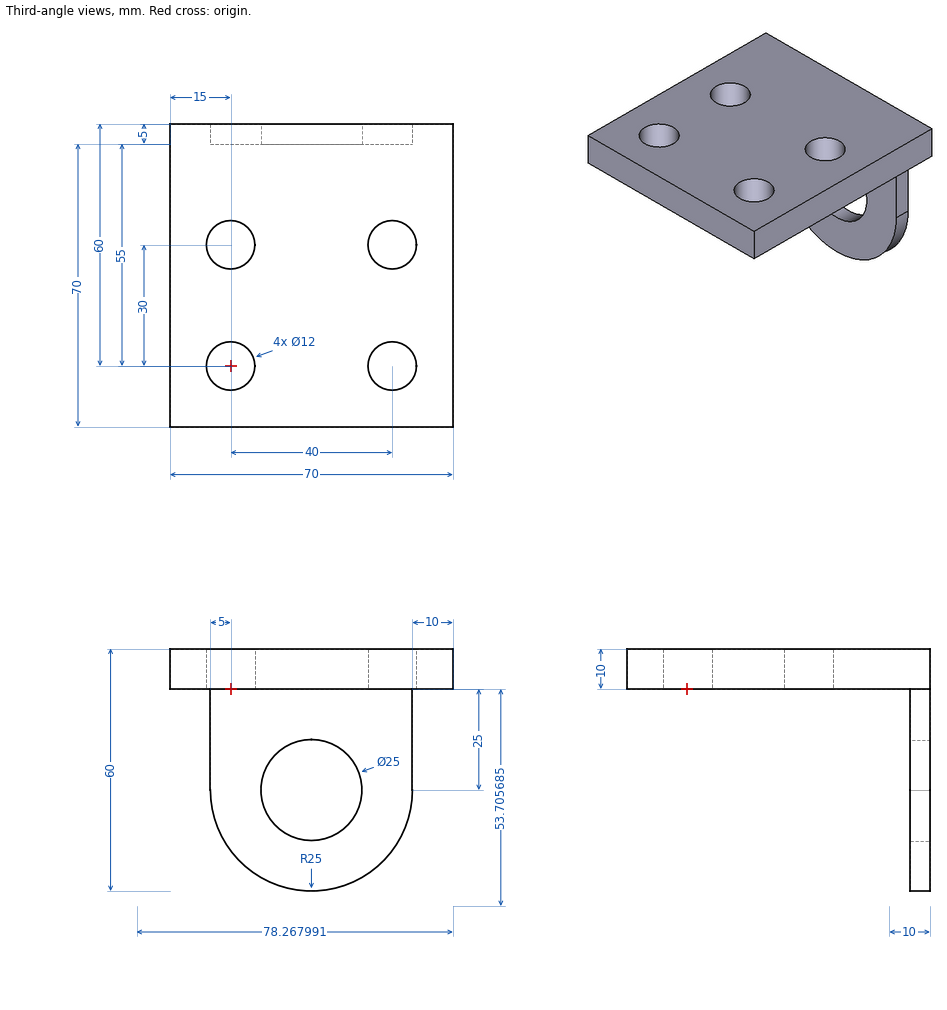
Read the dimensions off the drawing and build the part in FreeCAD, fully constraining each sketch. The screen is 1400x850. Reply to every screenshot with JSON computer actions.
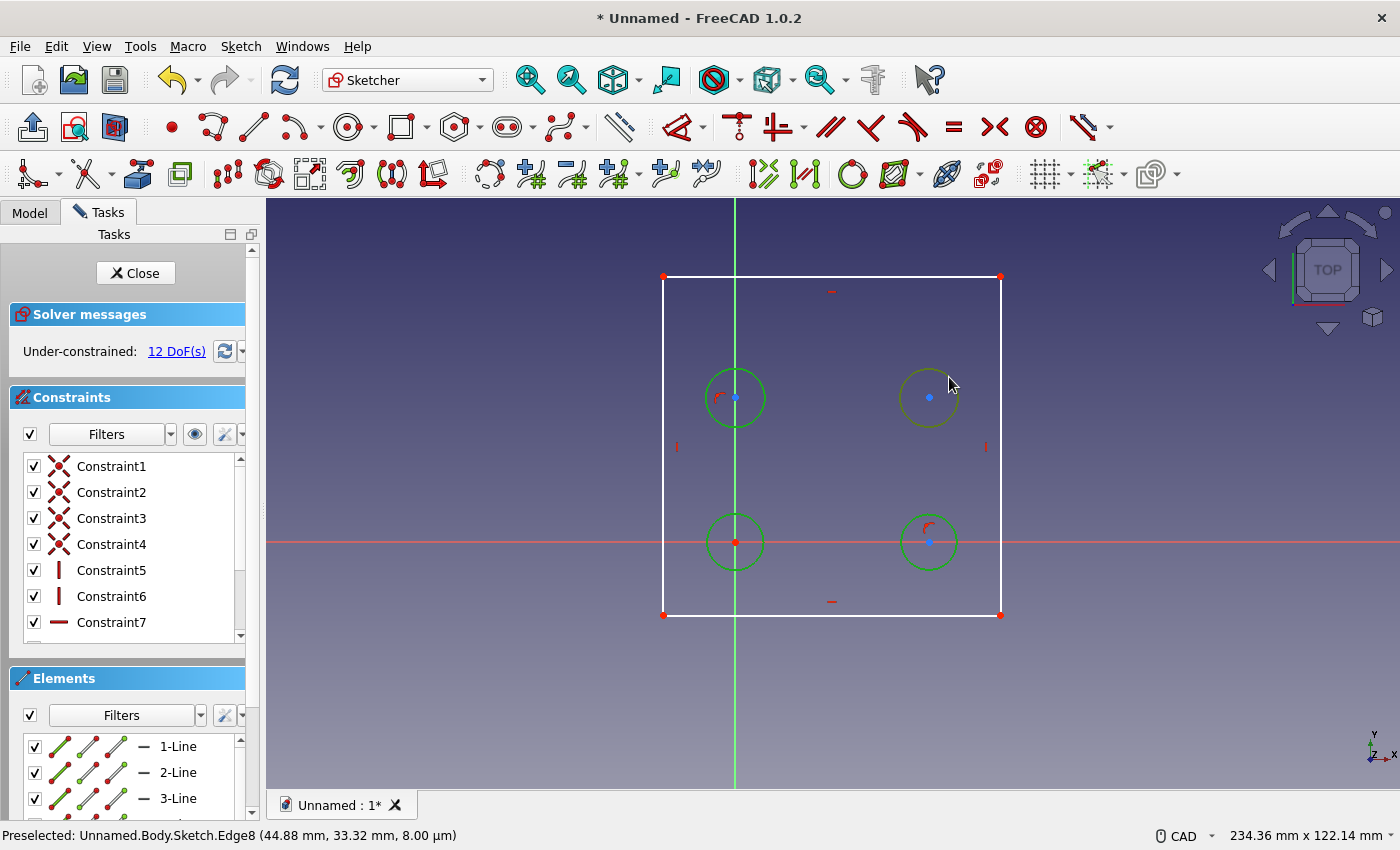
{"action": "left_click", "coordinate": [954, 128]}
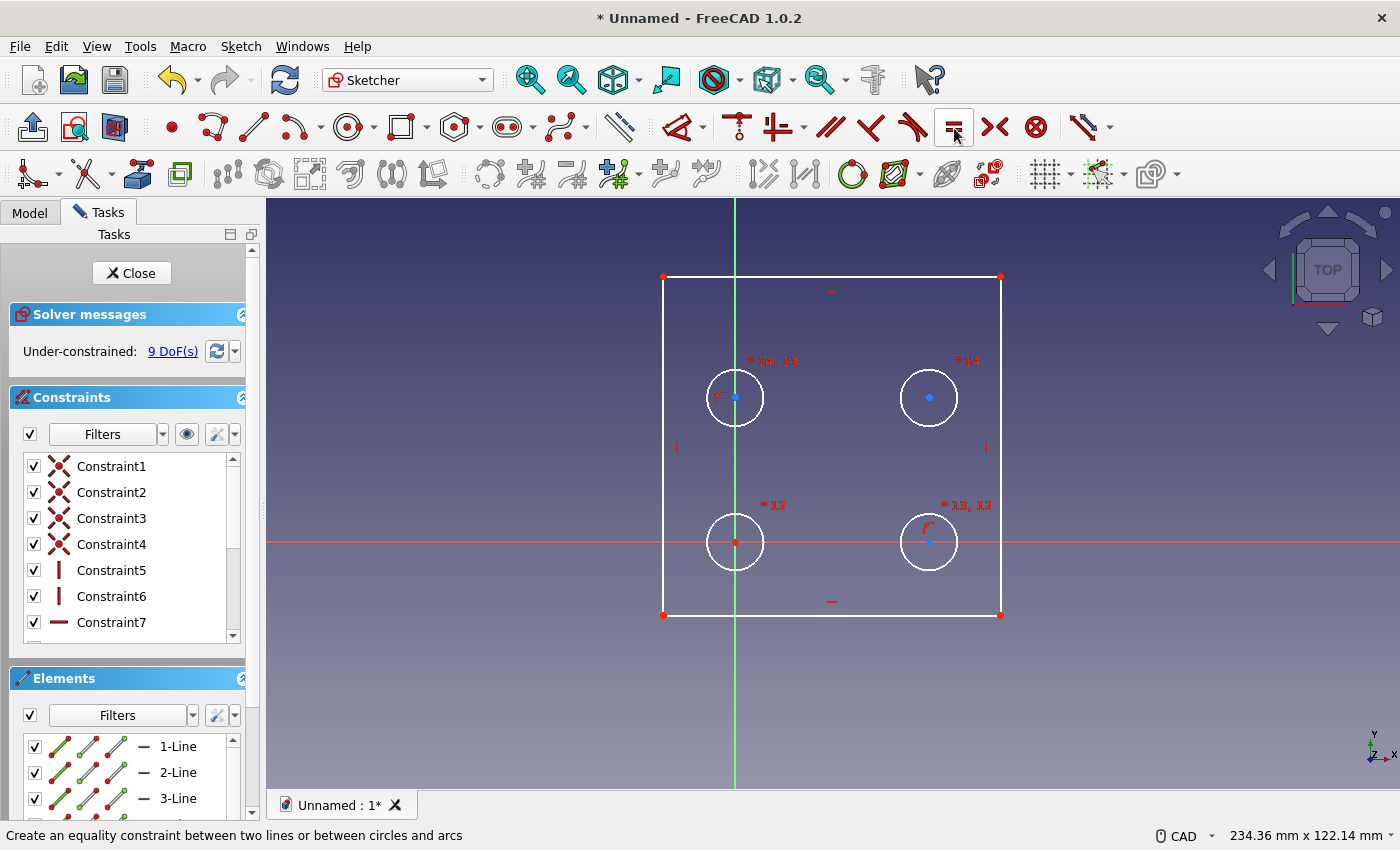
{"action": "left_click", "coordinate": [676, 128]}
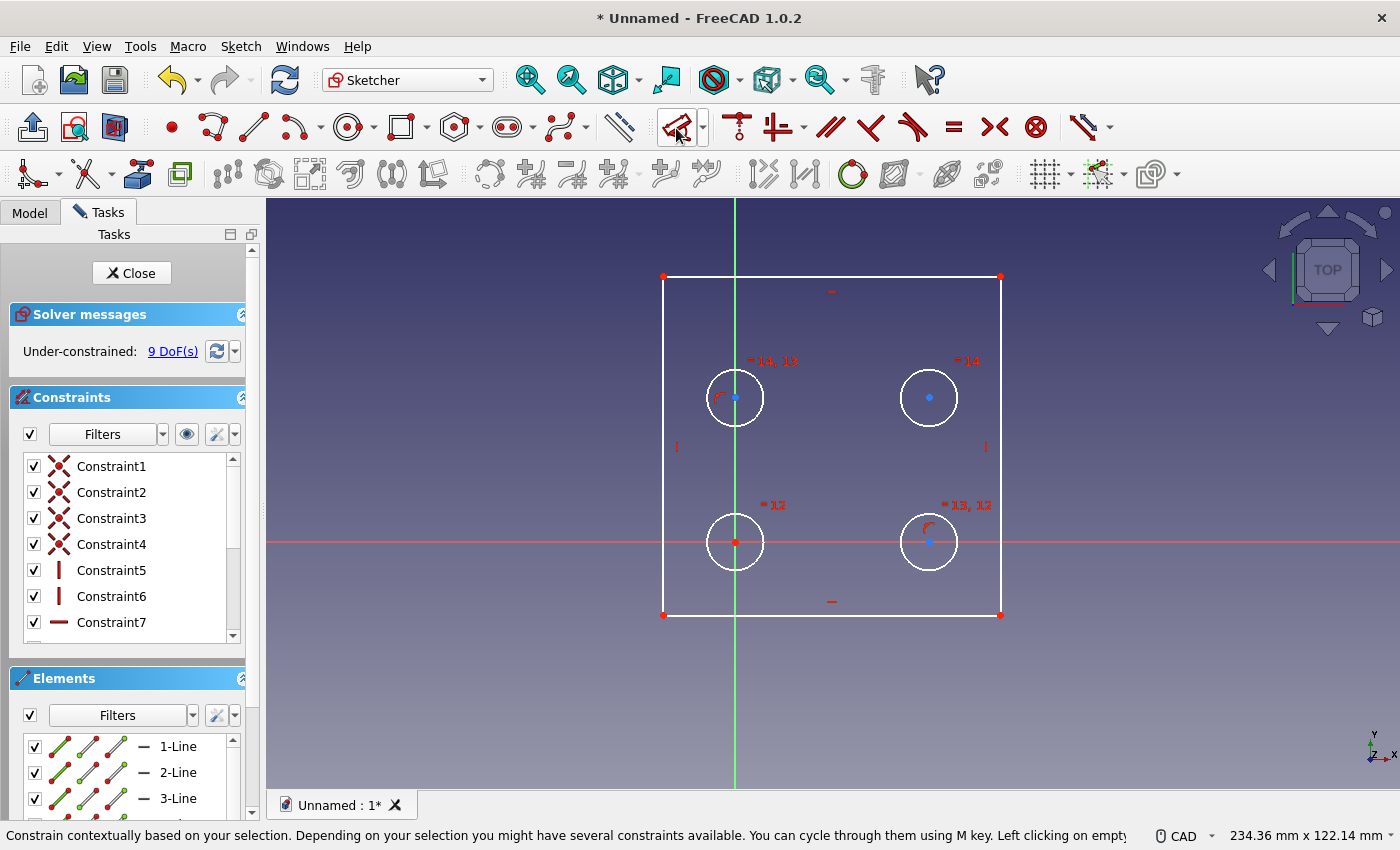
{"action": "left_click", "coordinate": [755, 522]}
{"action": "left_click", "coordinate": [777, 499]}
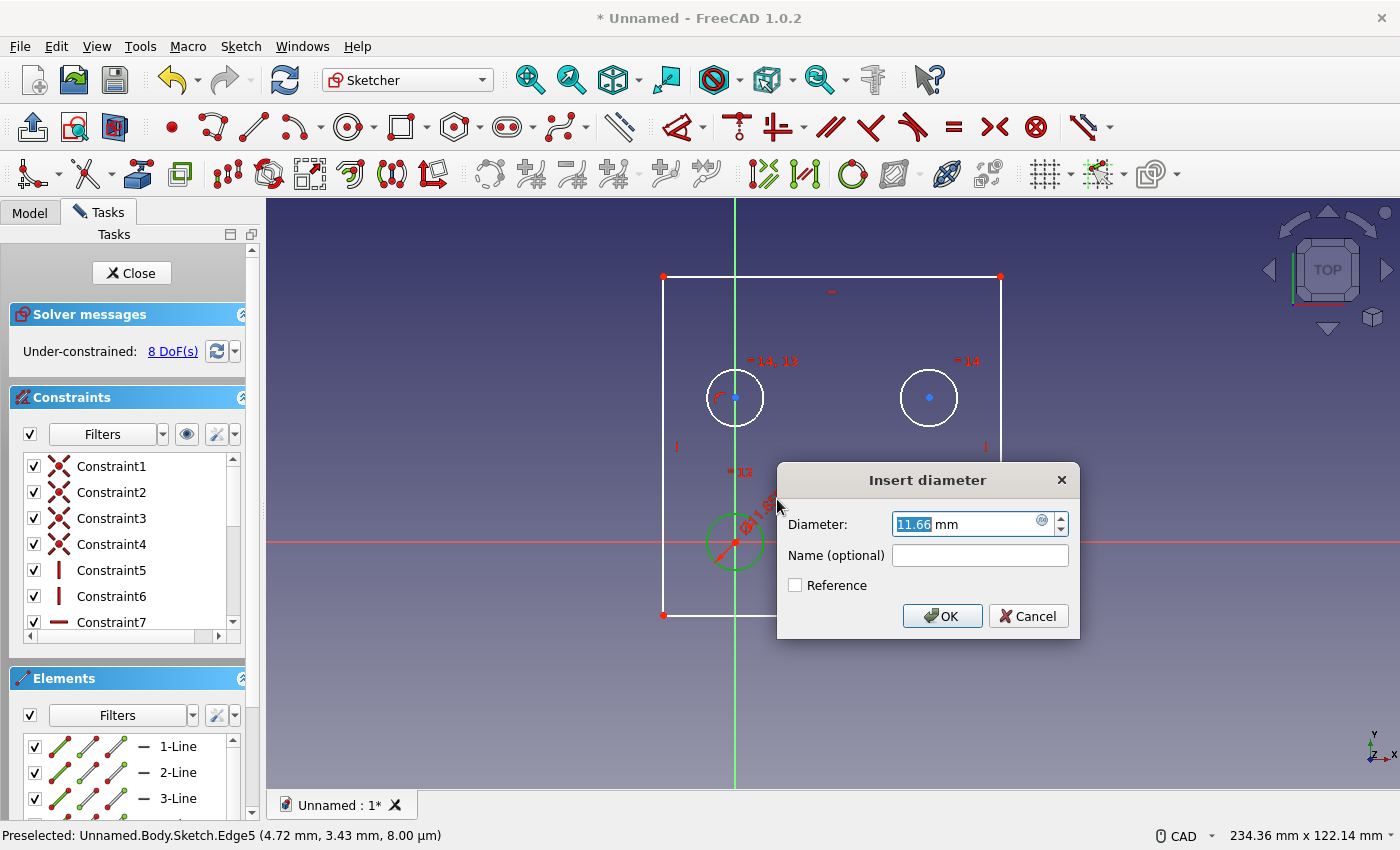
{"action": "type", "text": "12"}
{"action": "key", "text": "Return"}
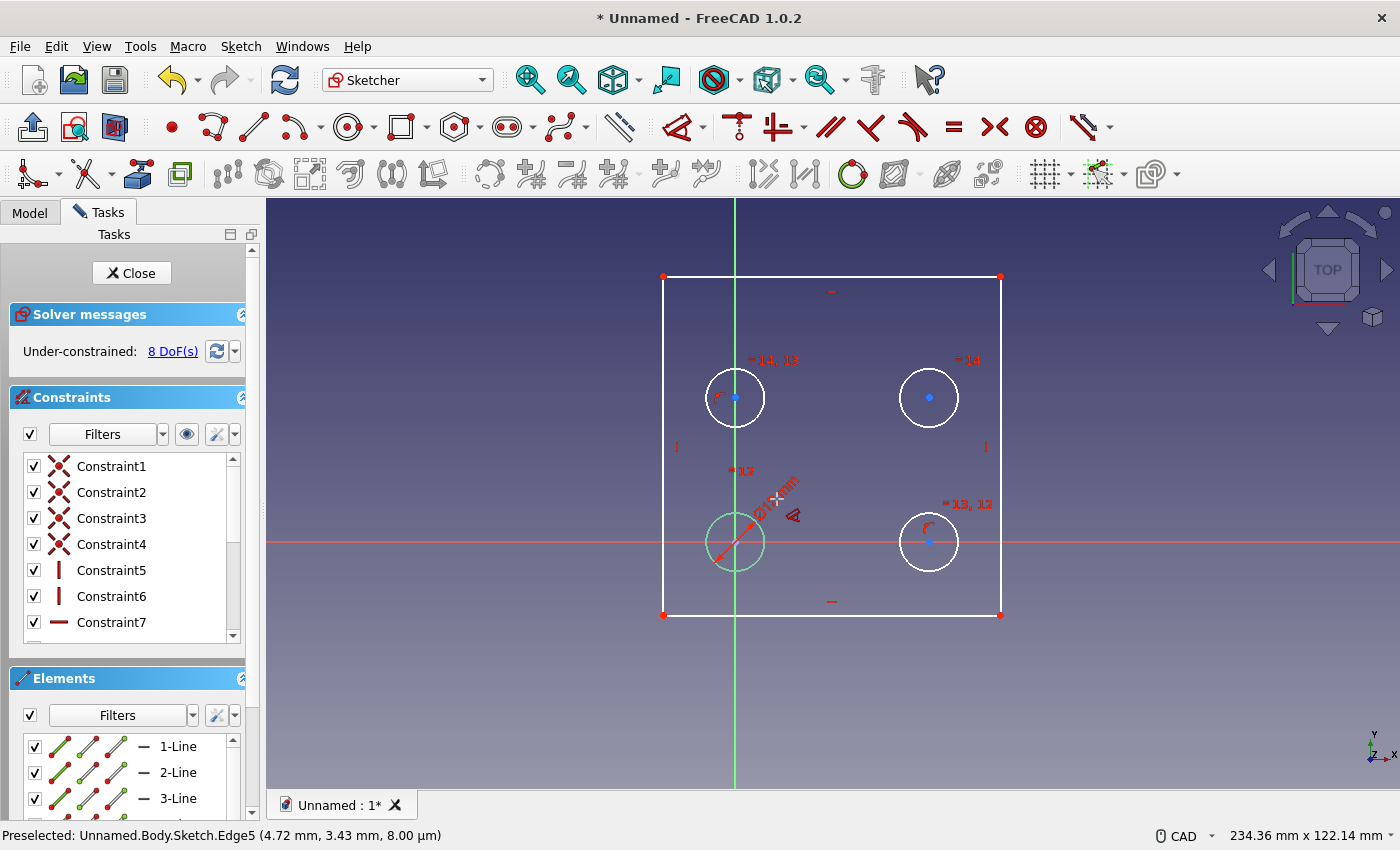
{"action": "left_click", "coordinate": [663, 379]}
{"action": "left_click", "coordinate": [629, 447]}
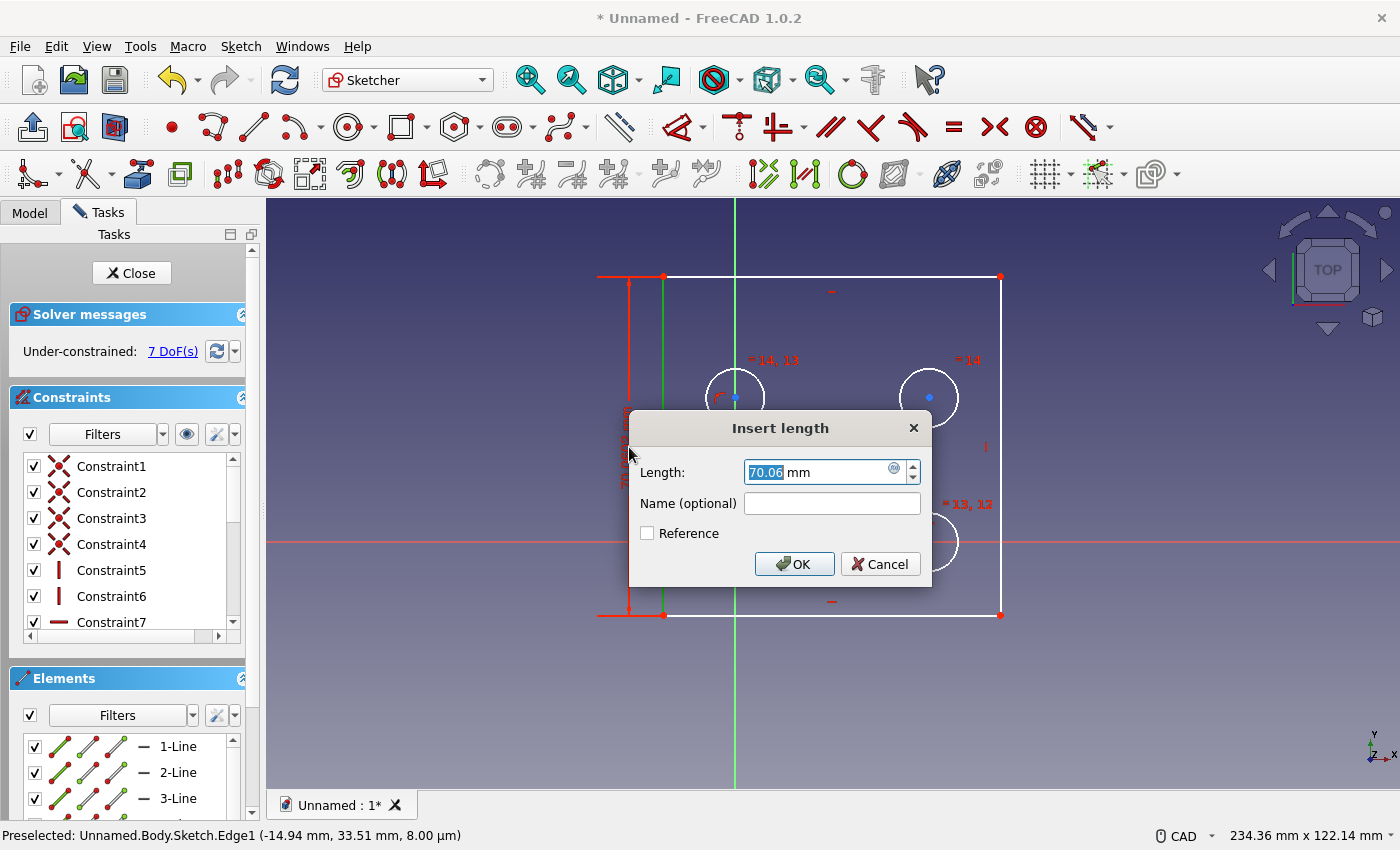
{"action": "type", "text": "70"}
{"action": "key", "text": "Return"}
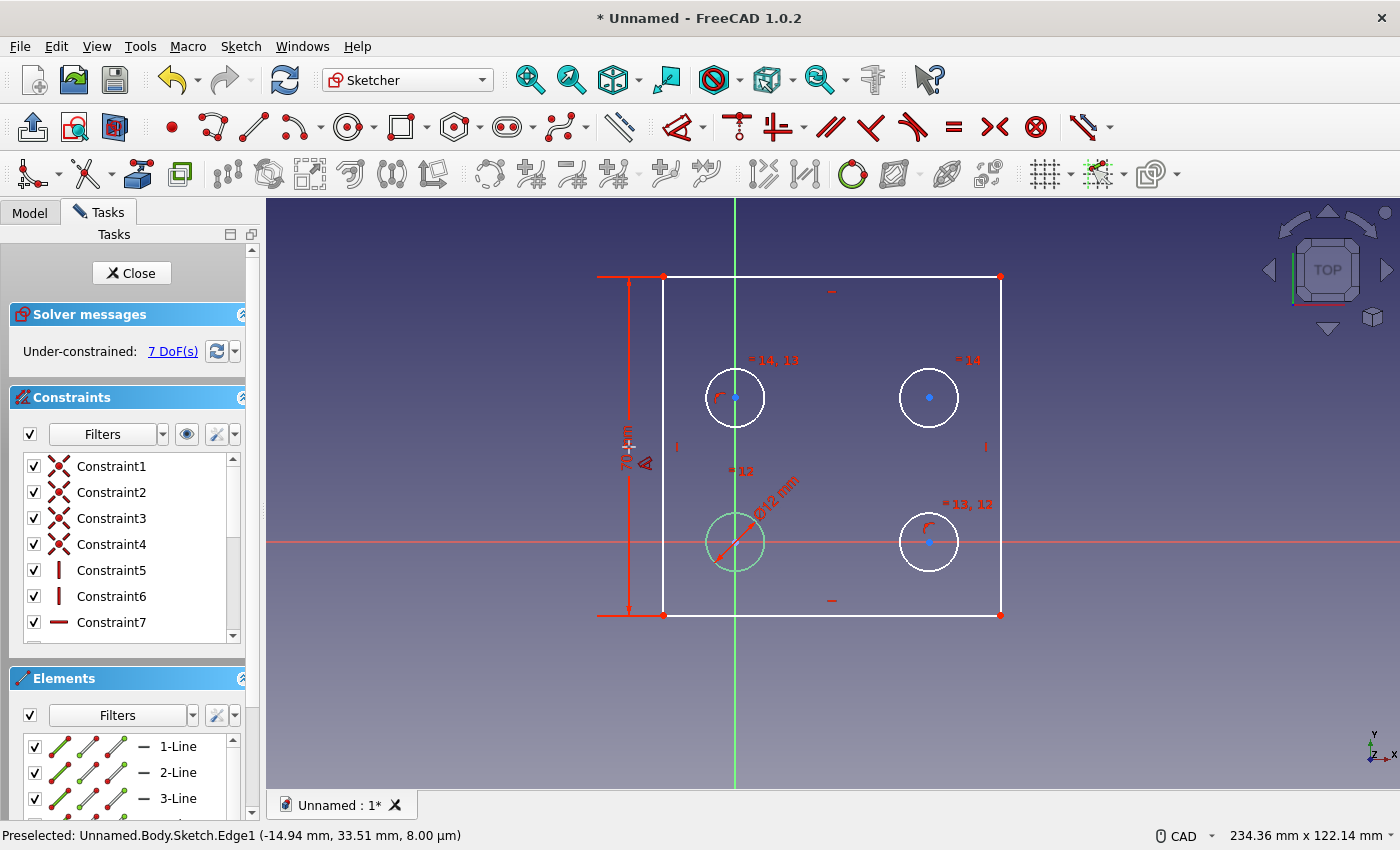
{"action": "left_click", "coordinate": [764, 616]}
{"action": "left_click", "coordinate": [832, 650]}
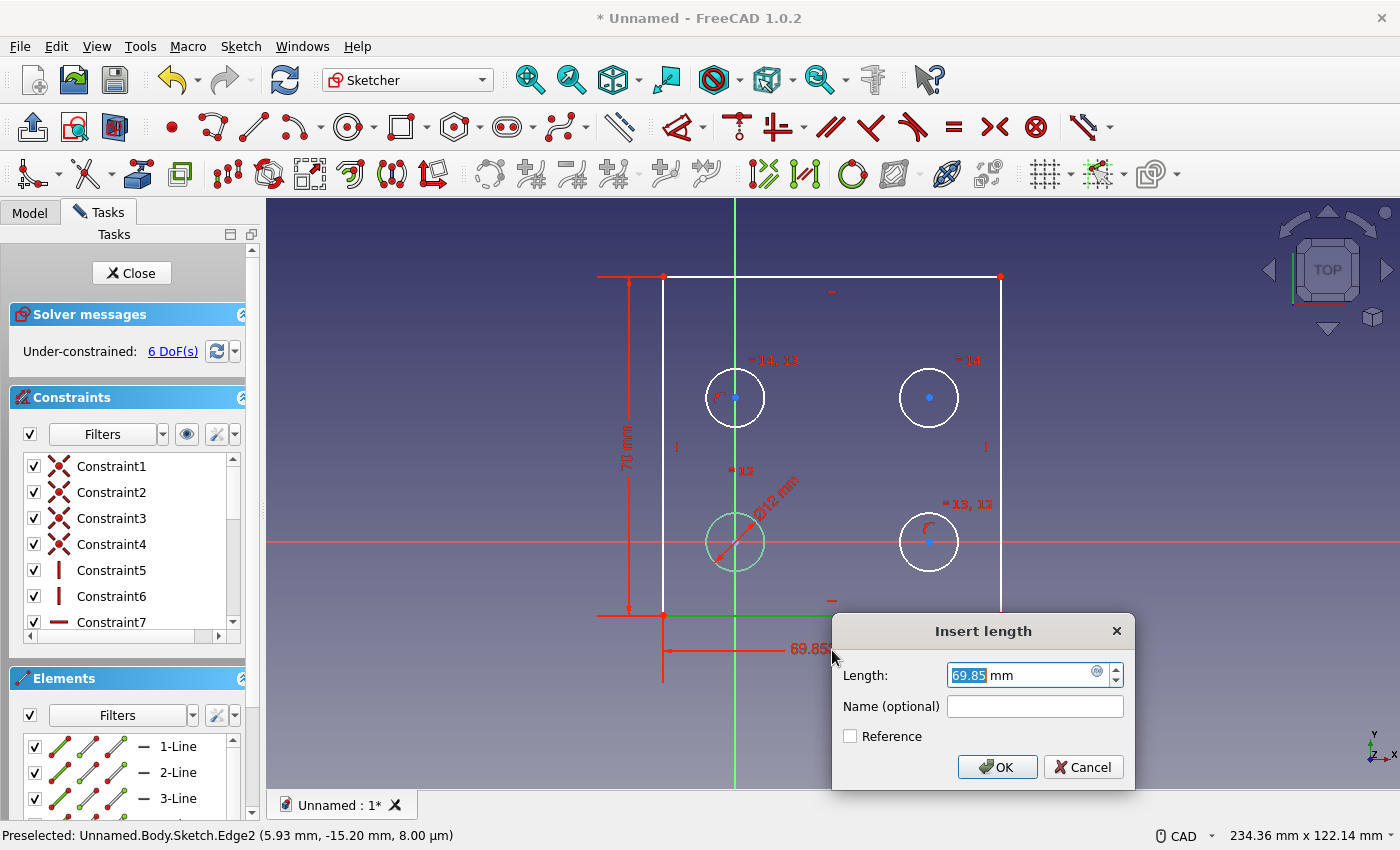
{"action": "type", "text": "70"}
{"action": "key", "text": "Return"}